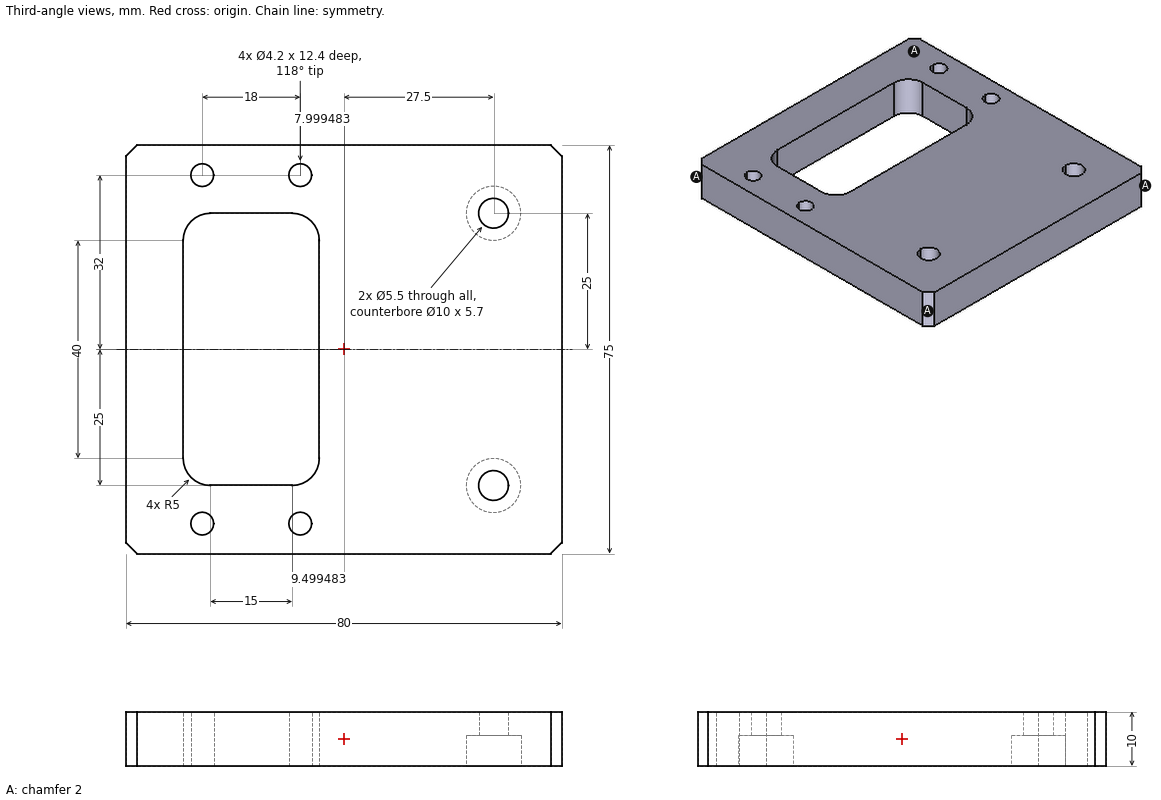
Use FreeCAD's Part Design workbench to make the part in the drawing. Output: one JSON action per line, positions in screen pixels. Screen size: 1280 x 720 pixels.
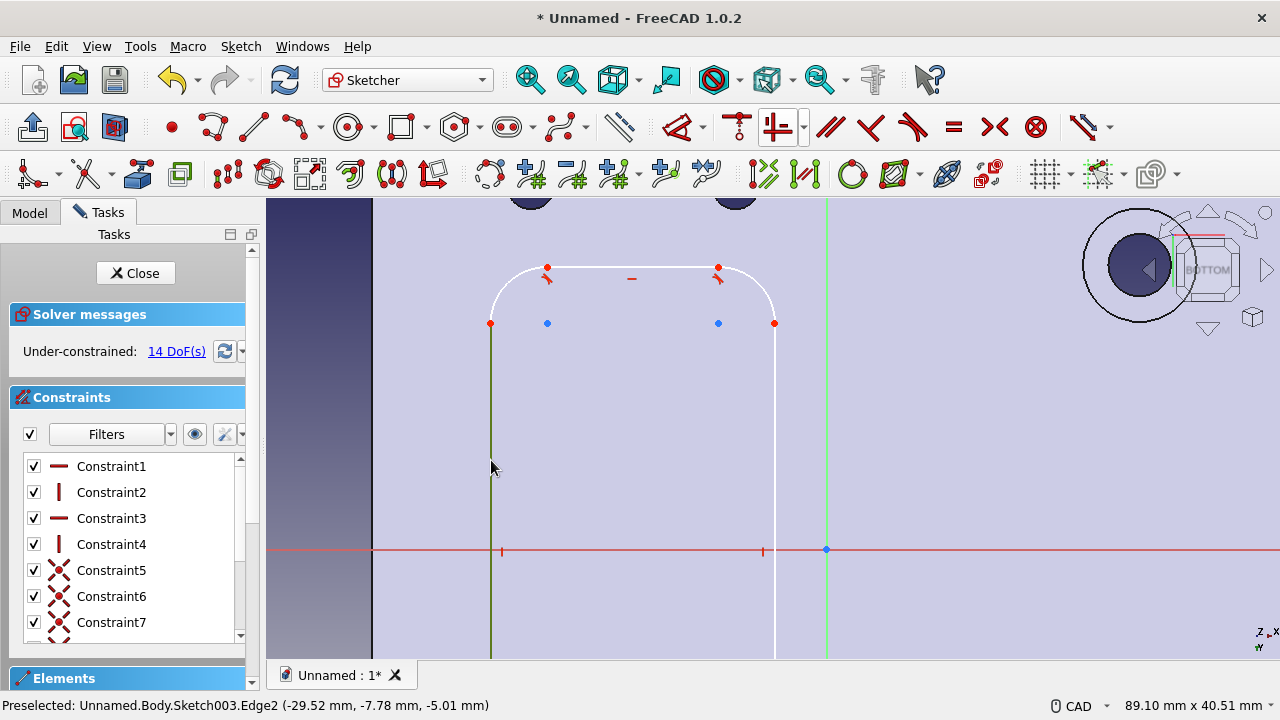
{"action": "left_click", "coordinate": [522, 273]}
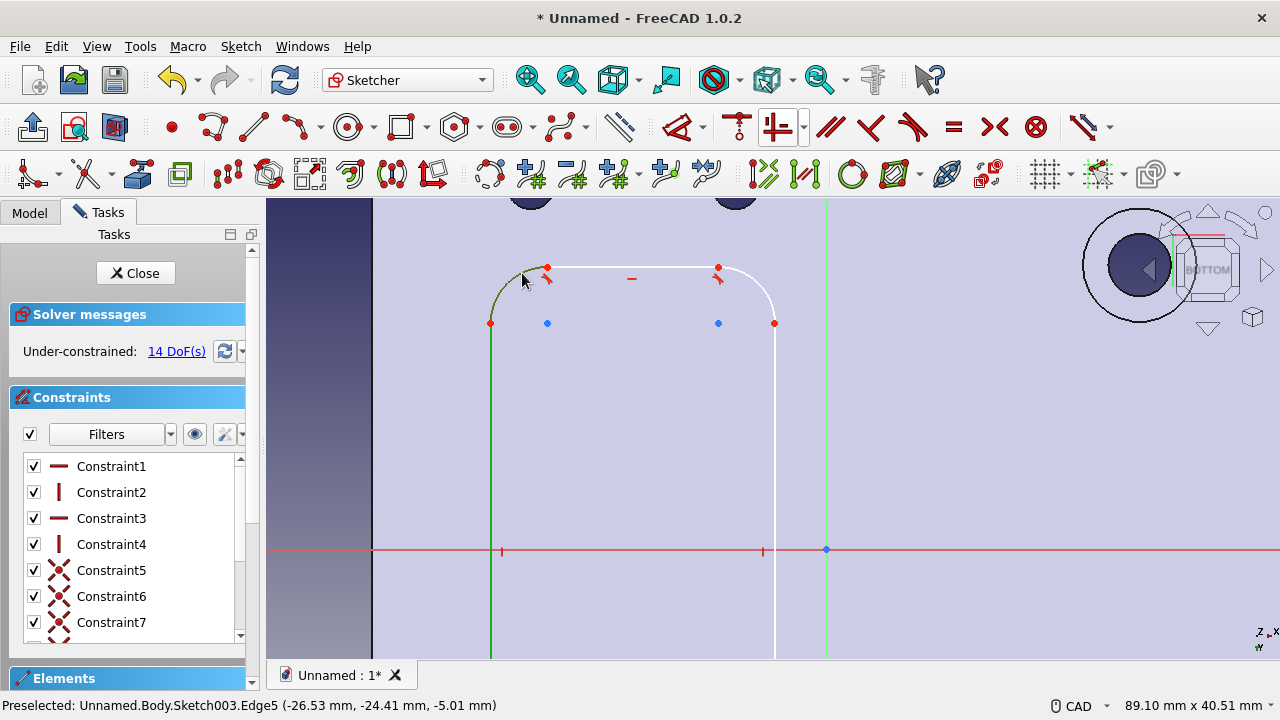
{"action": "left_click", "coordinate": [913, 128]}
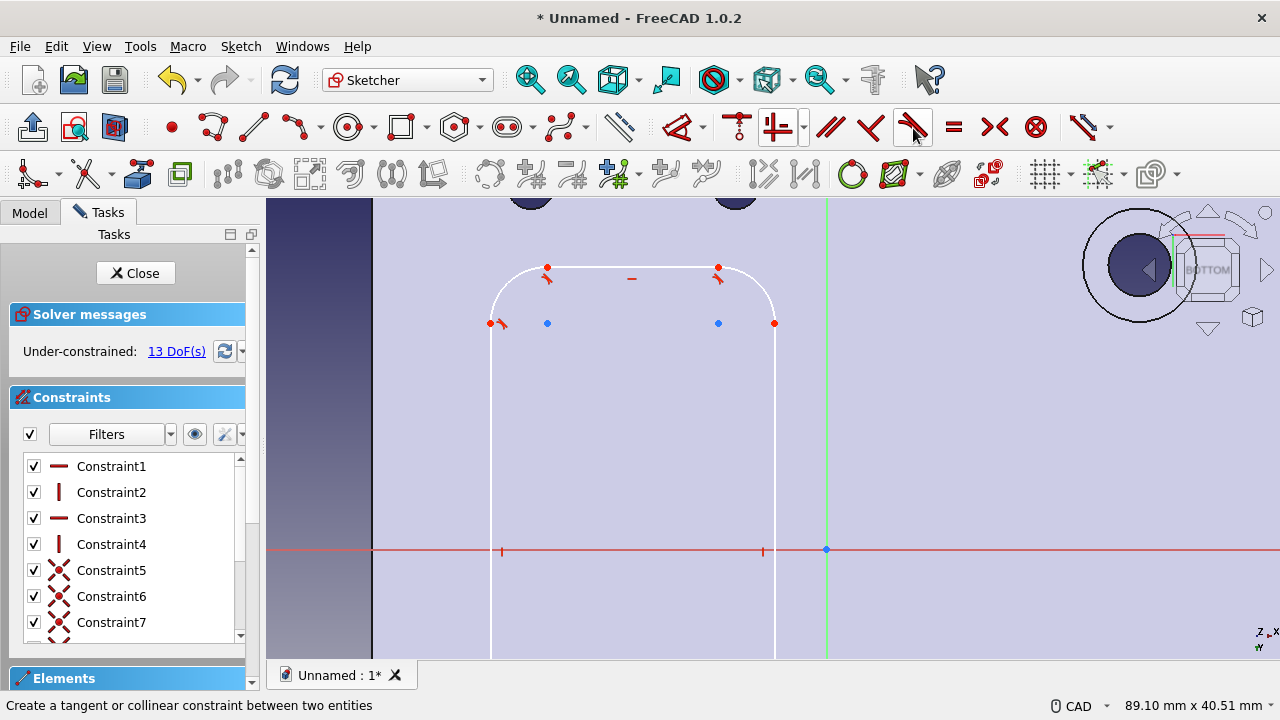
{"action": "left_click", "coordinate": [491, 460]}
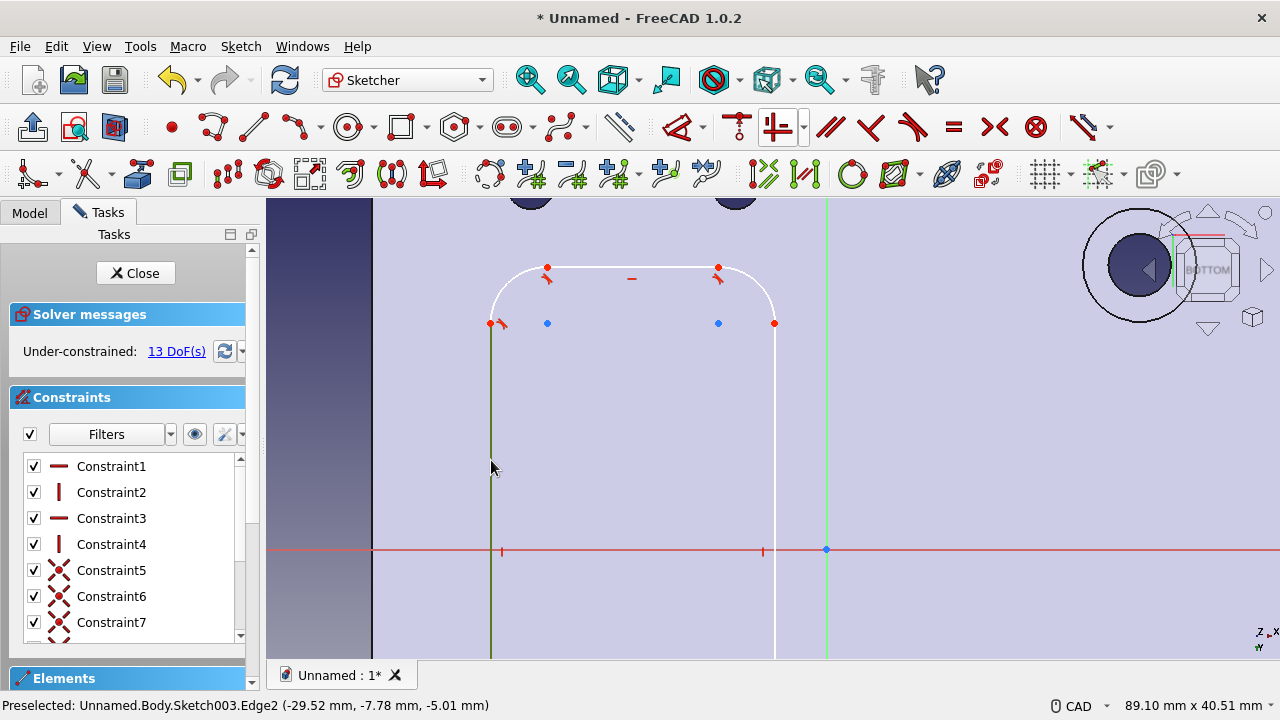
{"action": "scroll", "coordinate": [760, 281], "scroll_direction": "down", "scroll_amount": 3}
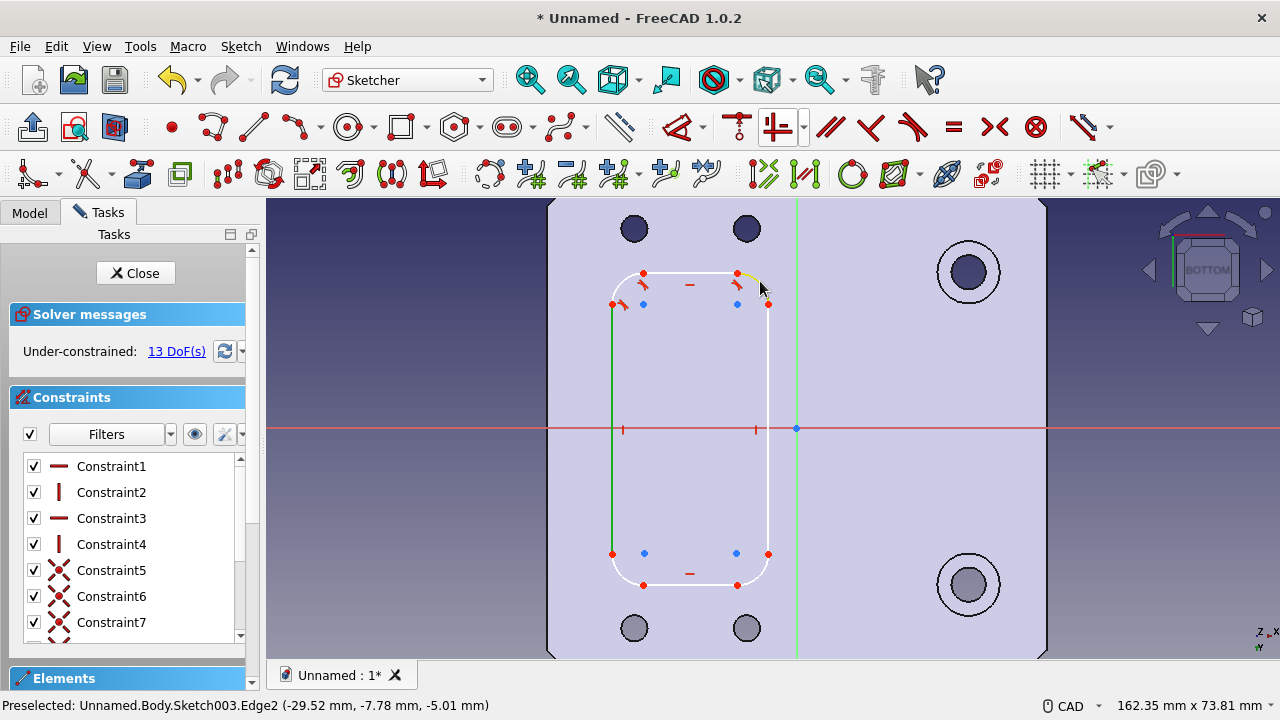
{"action": "left_click", "coordinate": [616, 568]}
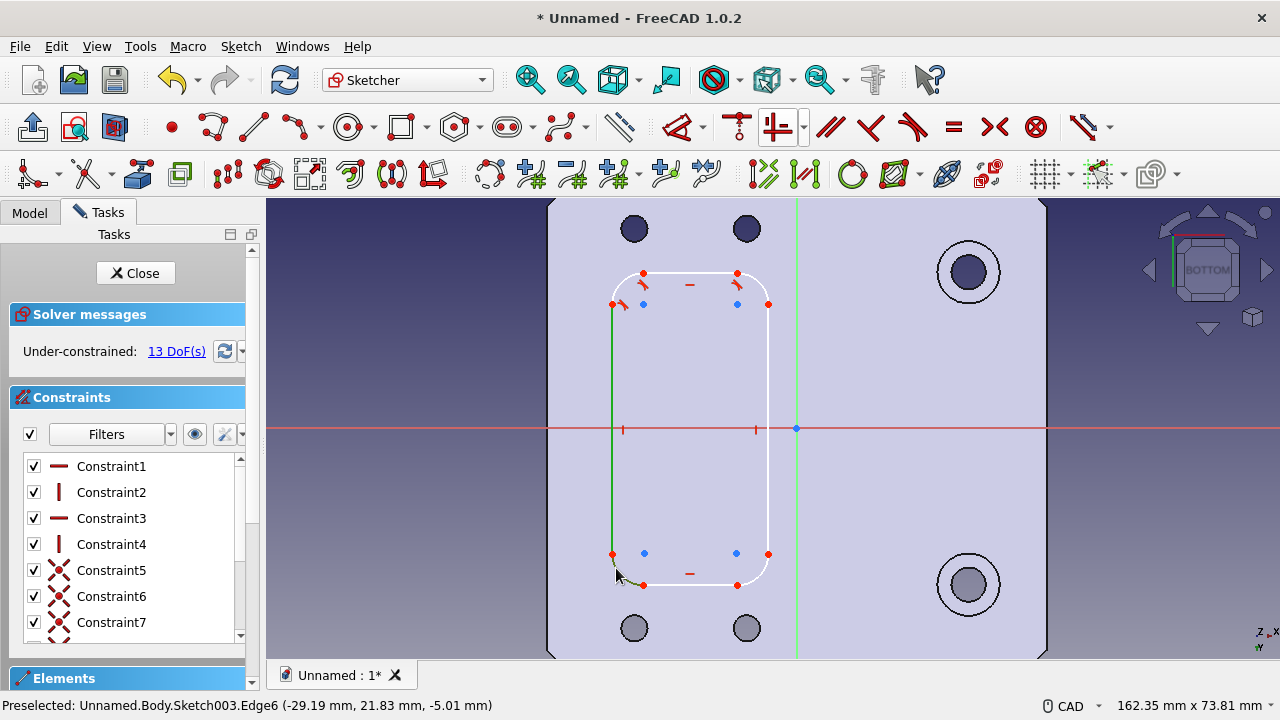
{"action": "key", "text": "t"}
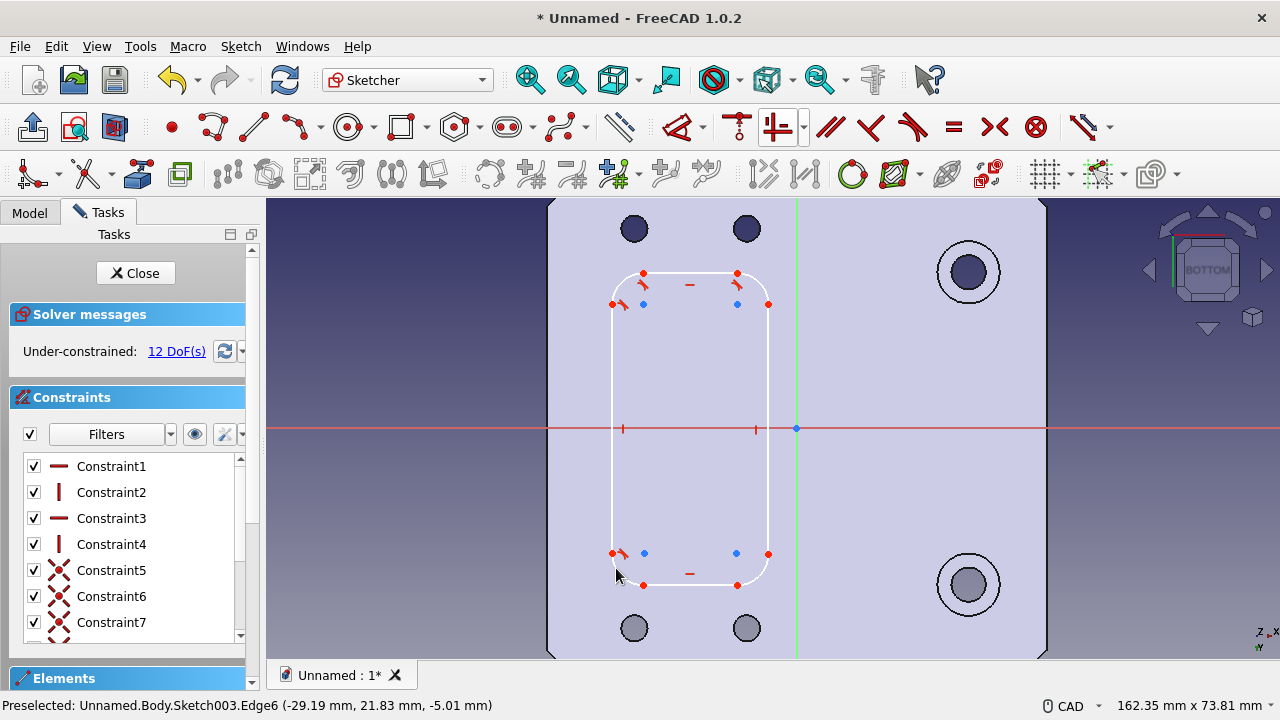
{"action": "left_click", "coordinate": [672, 585]}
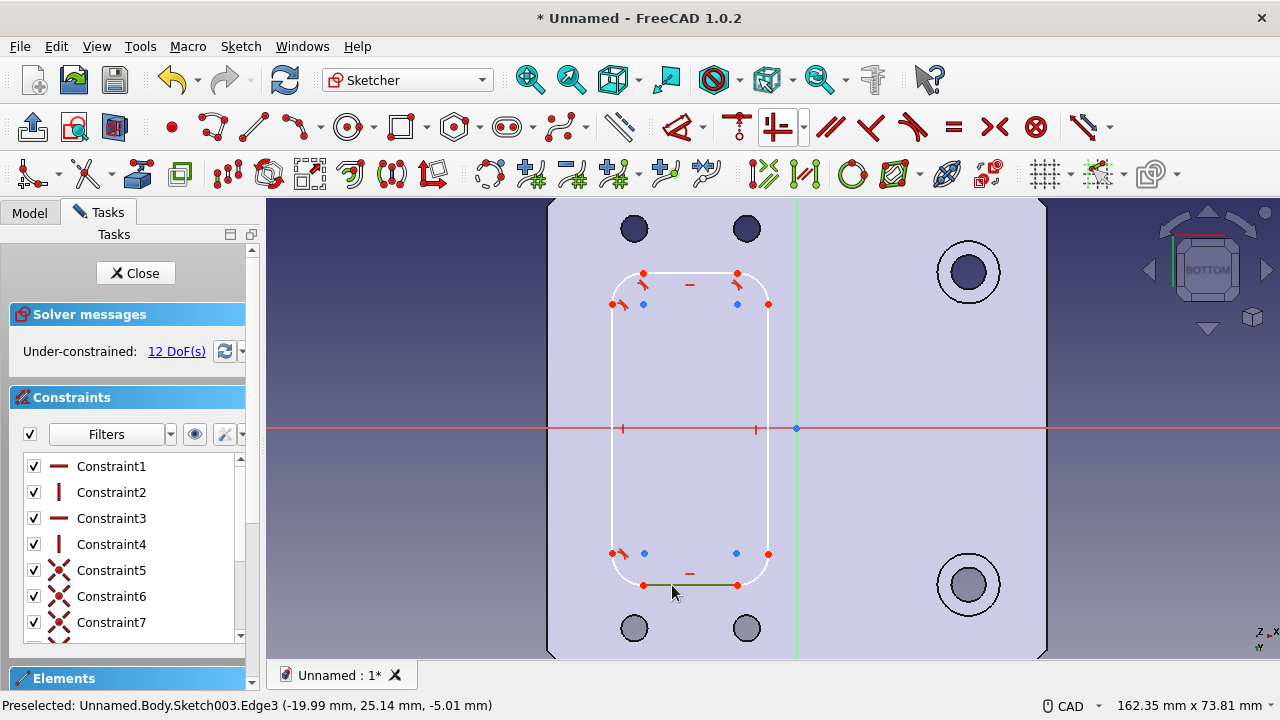
{"action": "left_click", "coordinate": [616, 568]}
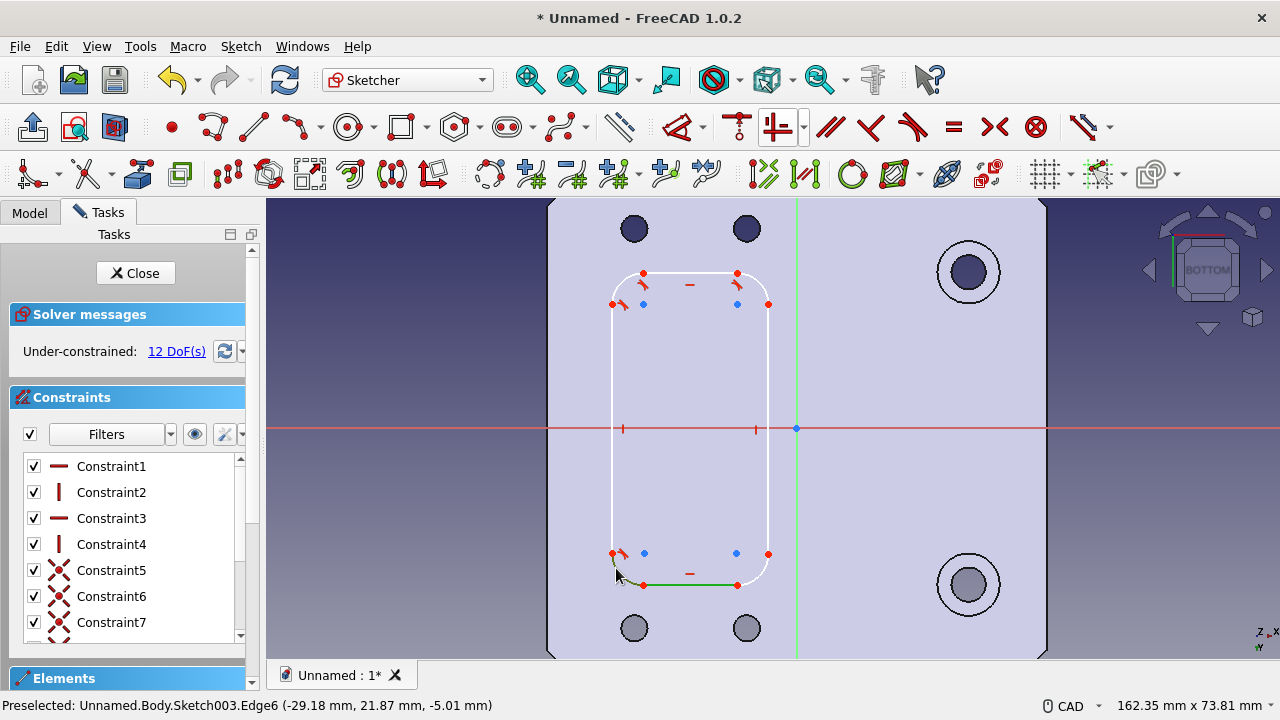
{"action": "key", "text": "t"}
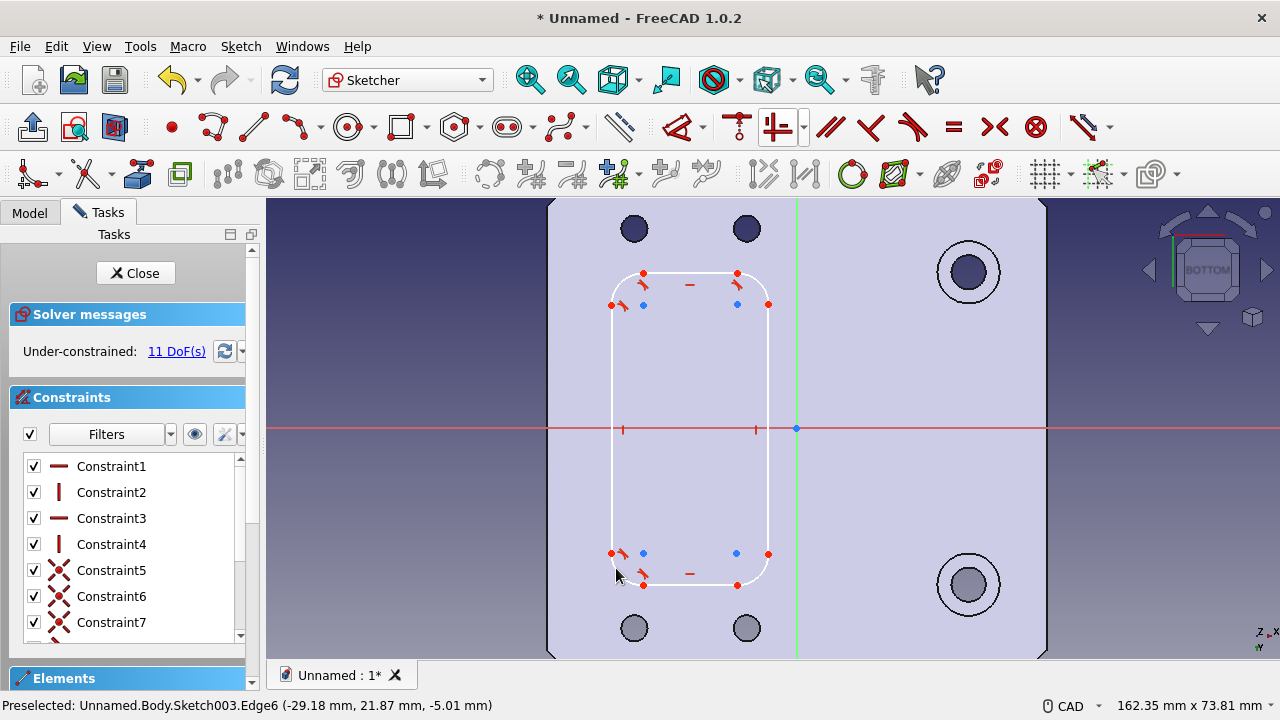
{"action": "left_click", "coordinate": [672, 585]}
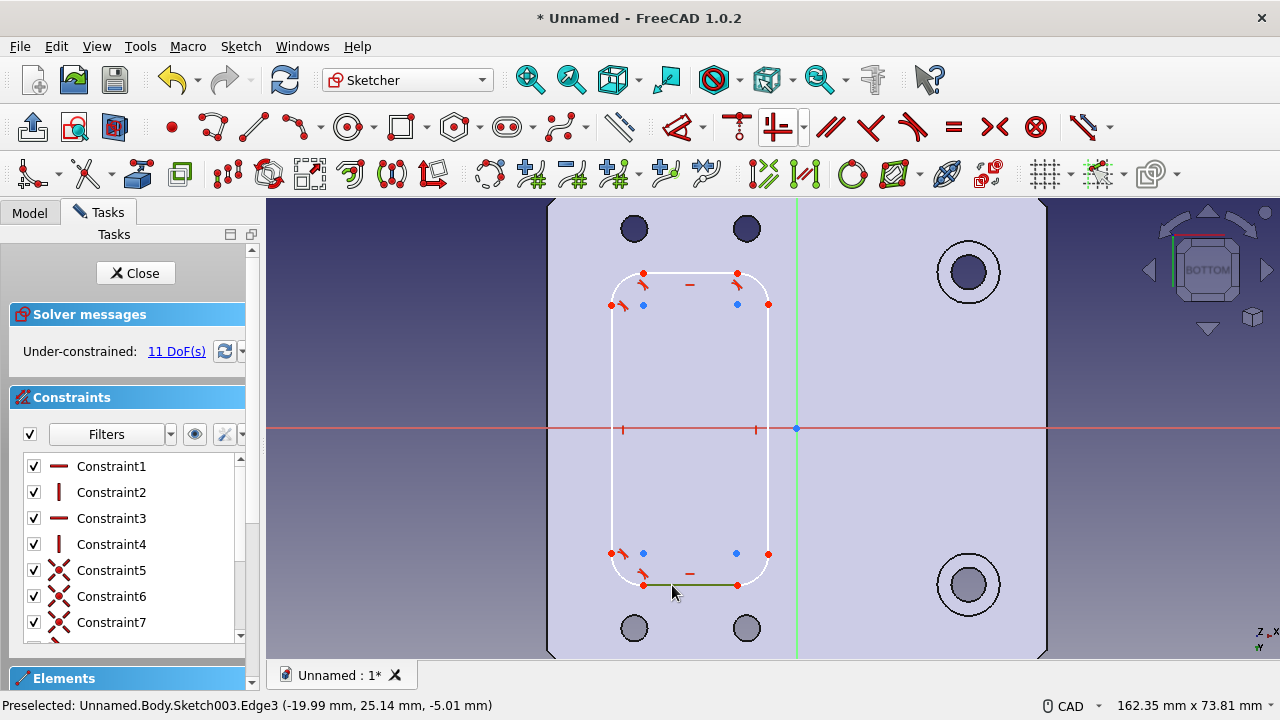
{"action": "left_click", "coordinate": [751, 582]}